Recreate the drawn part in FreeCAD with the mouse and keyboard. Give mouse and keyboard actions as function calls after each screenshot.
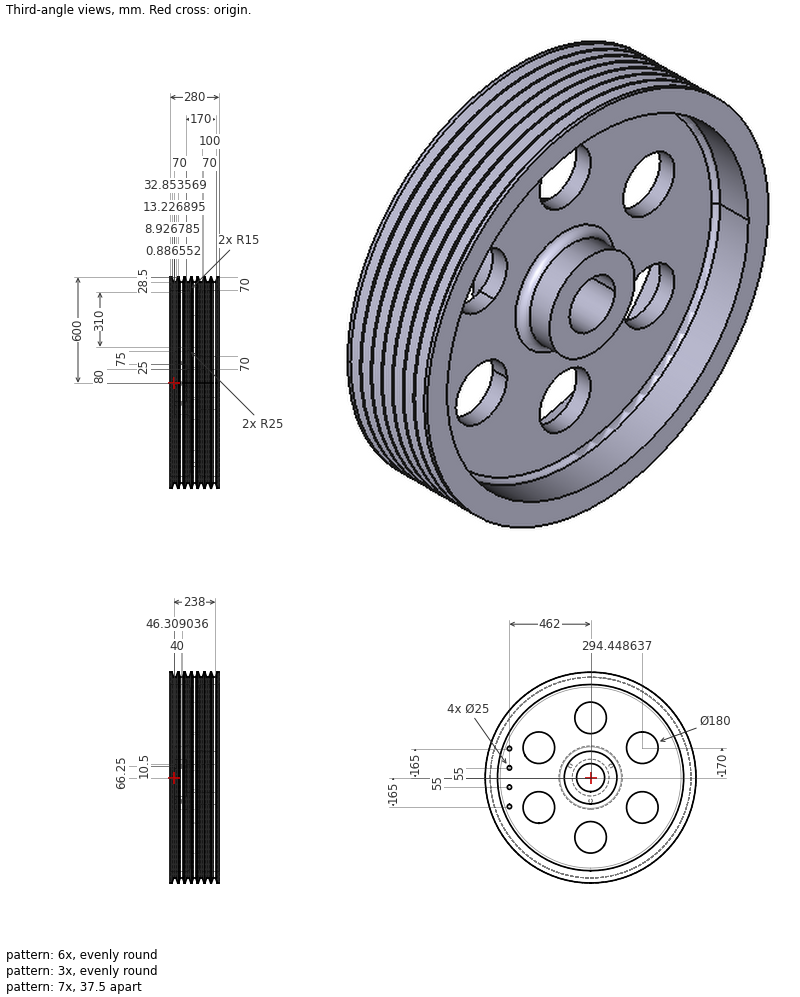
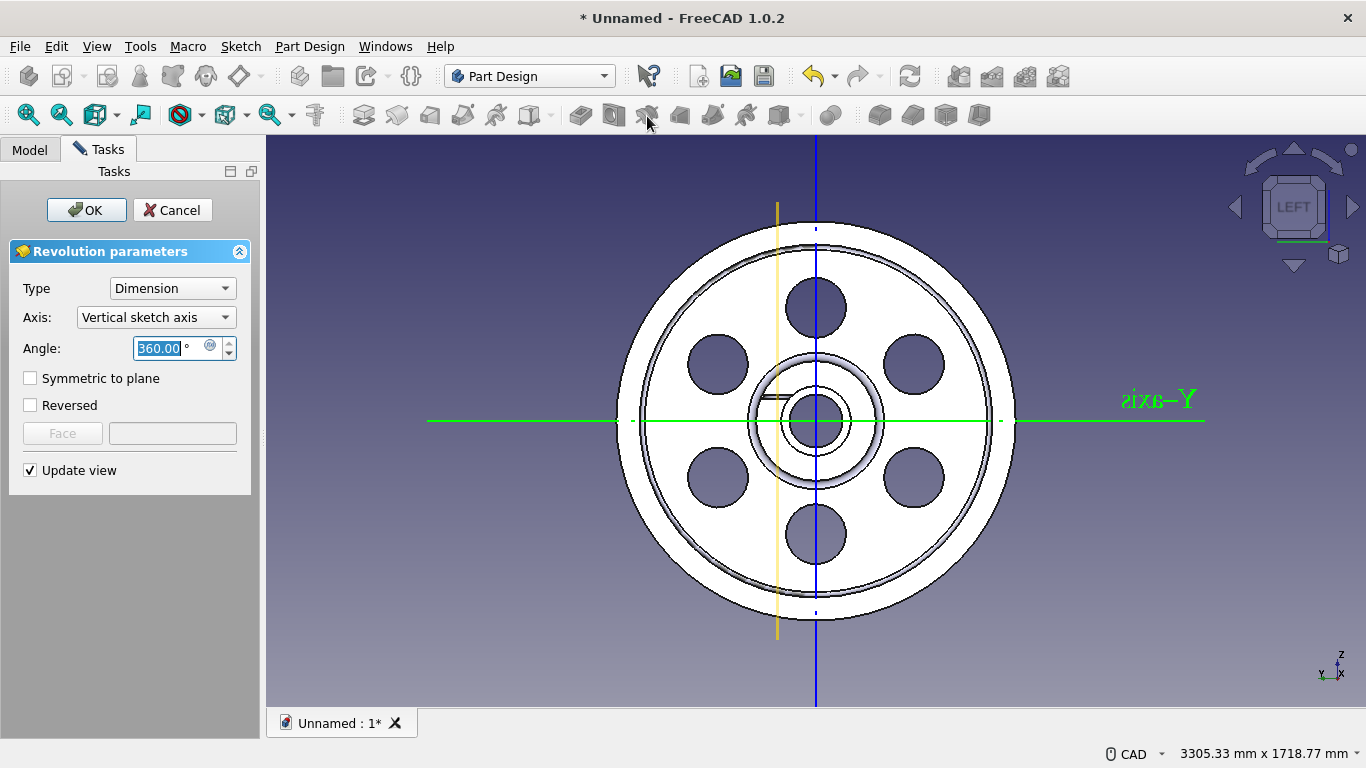
click(157, 318)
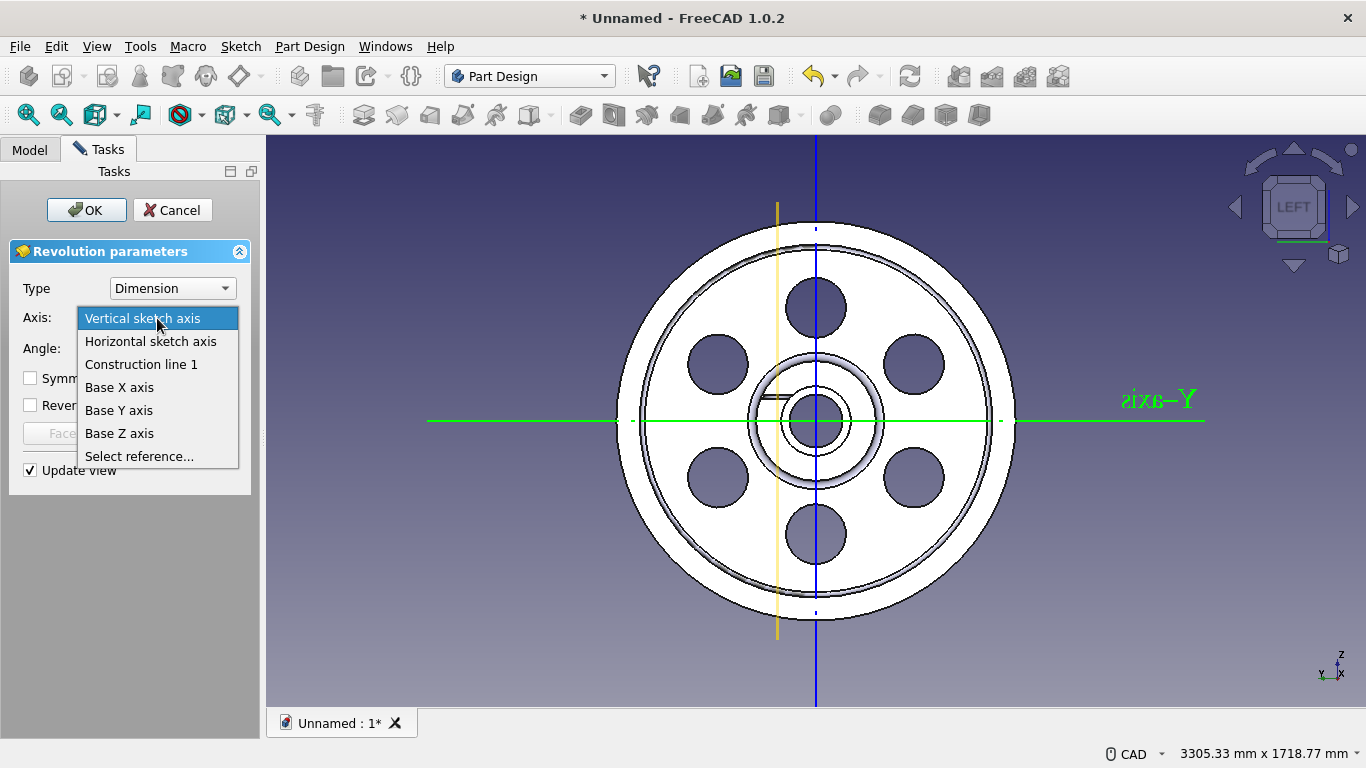
click(156, 364)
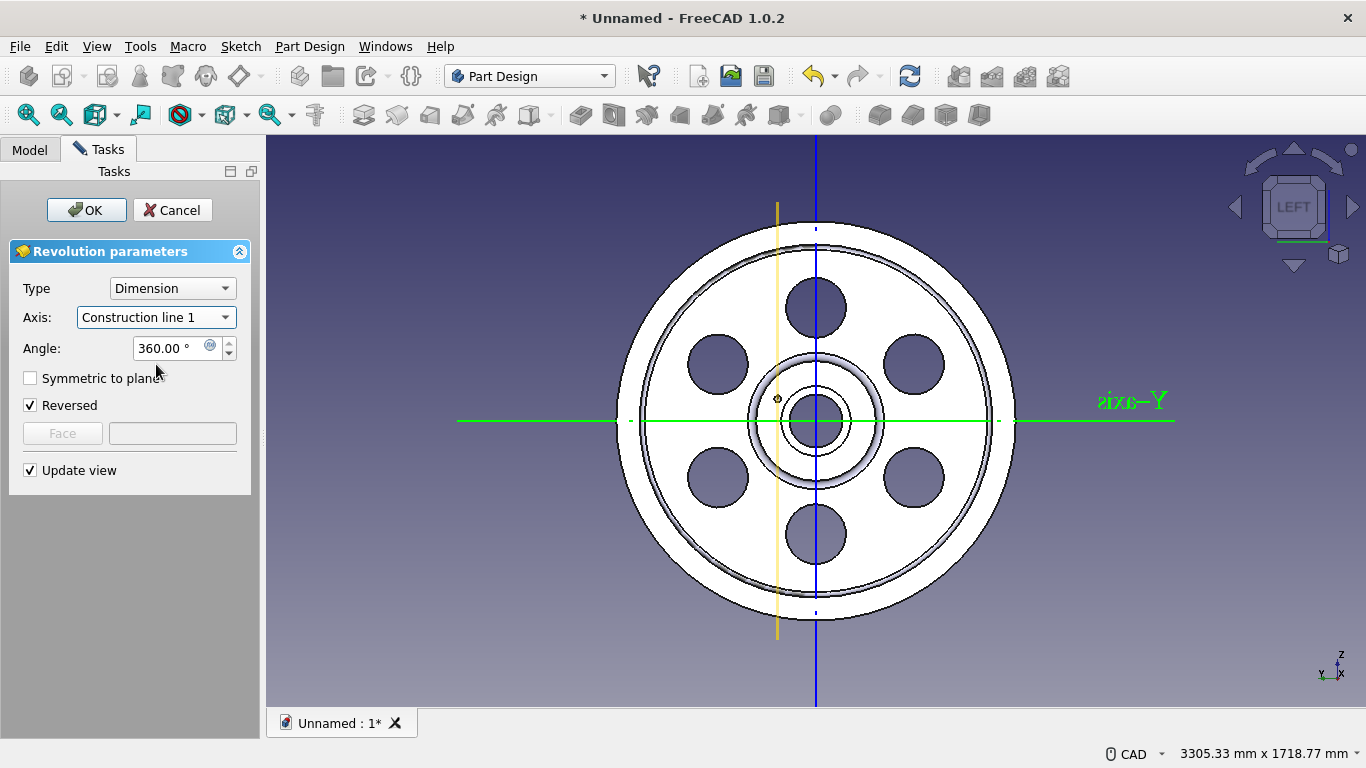
click(87, 210)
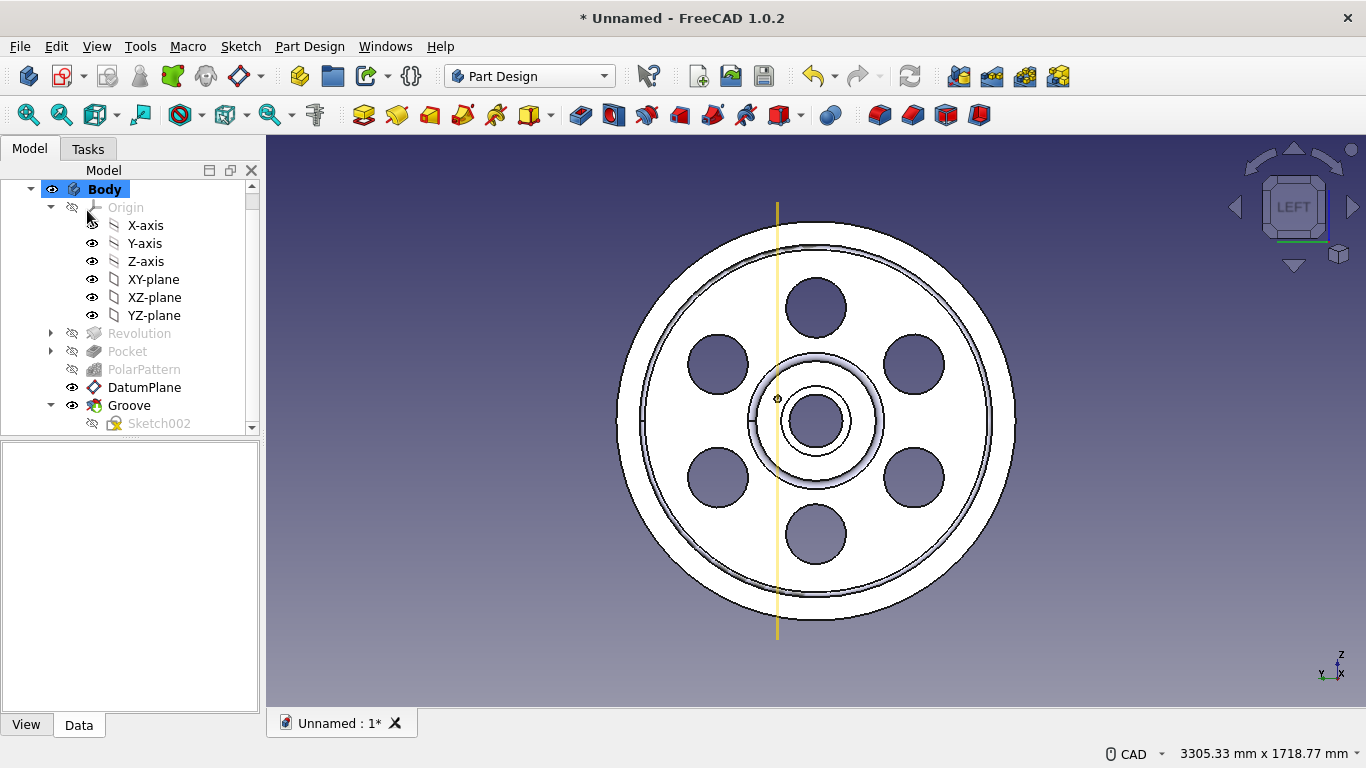
click(117, 387)
key(space)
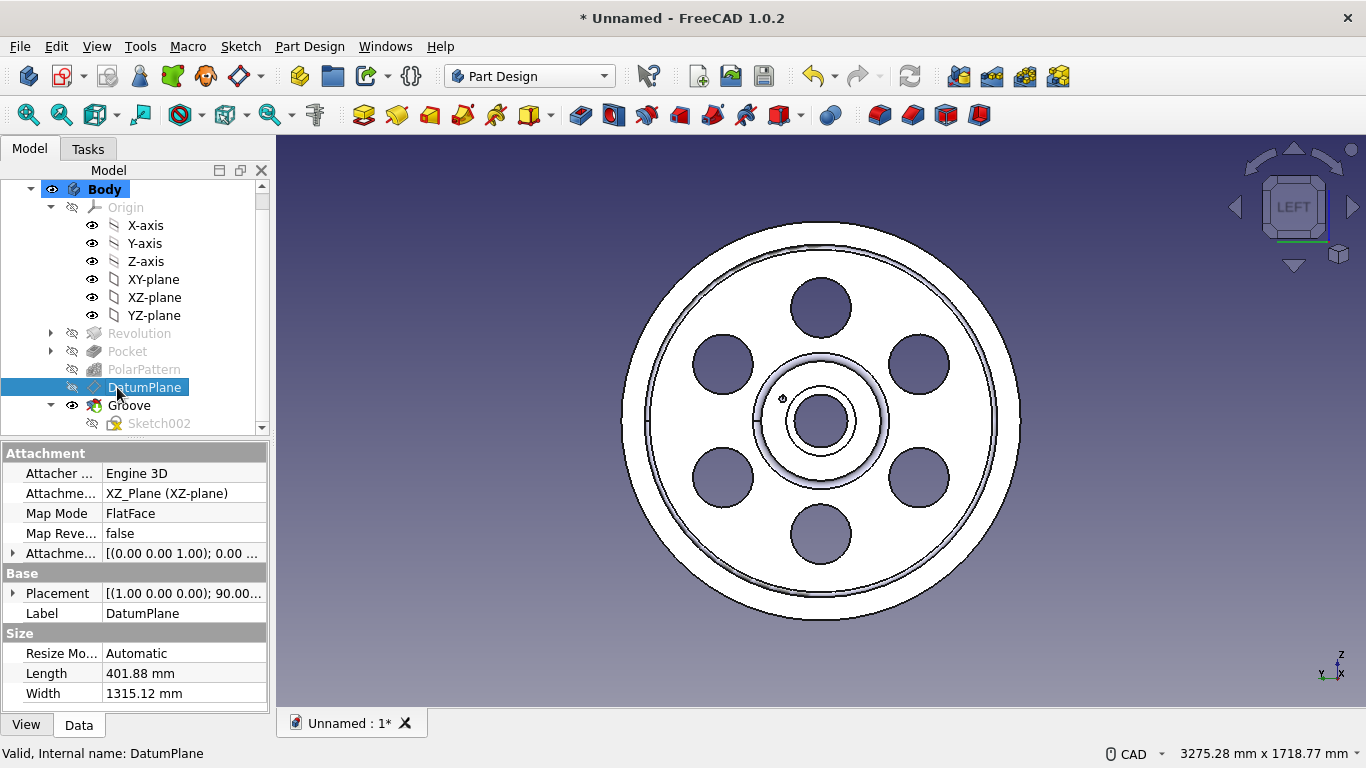
click(117, 405)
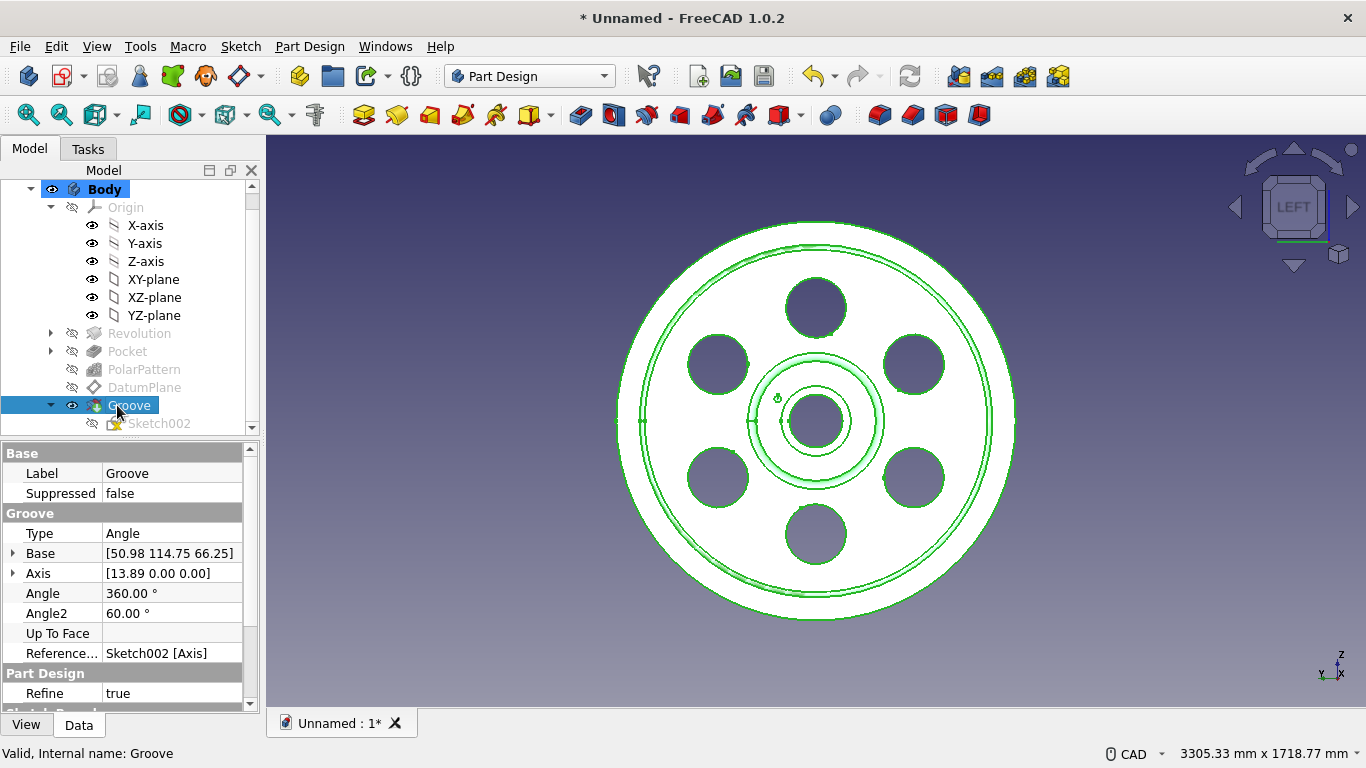
click(1025, 76)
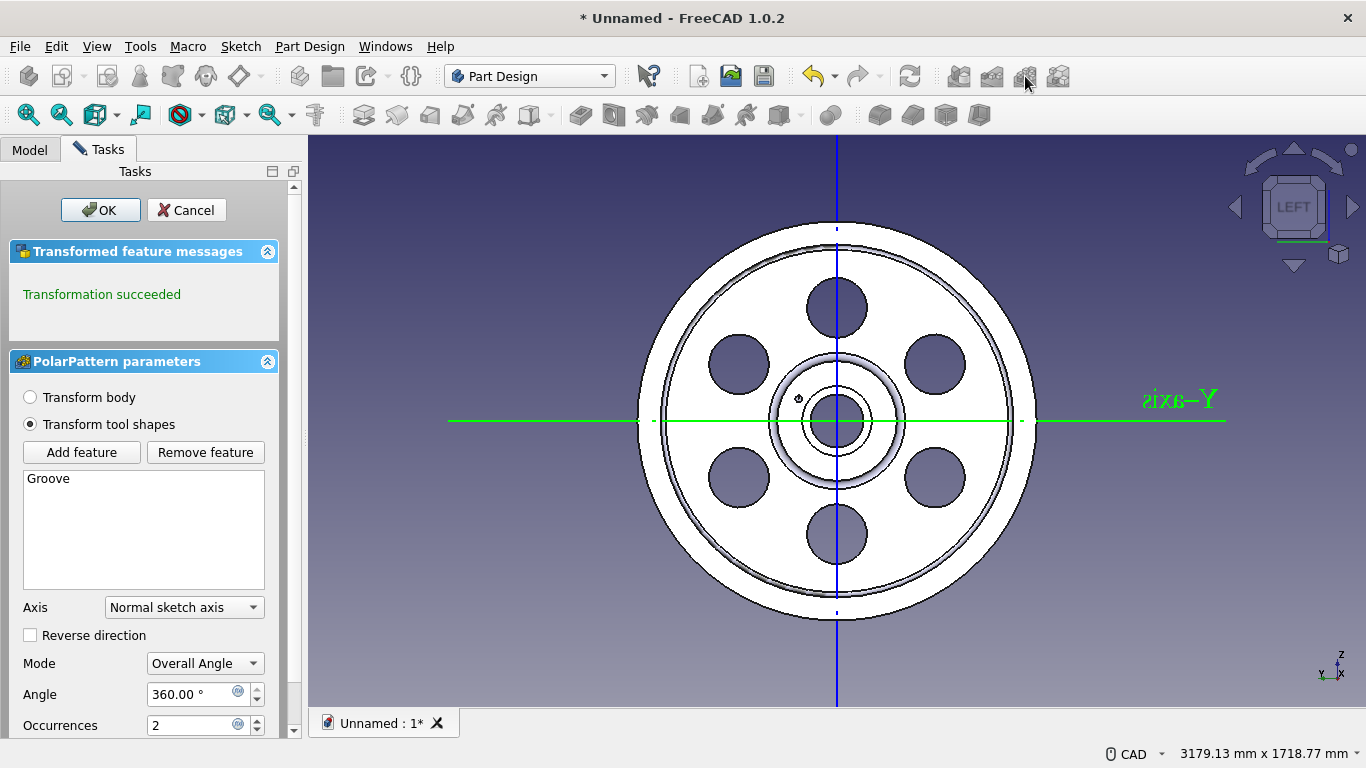
click(185, 608)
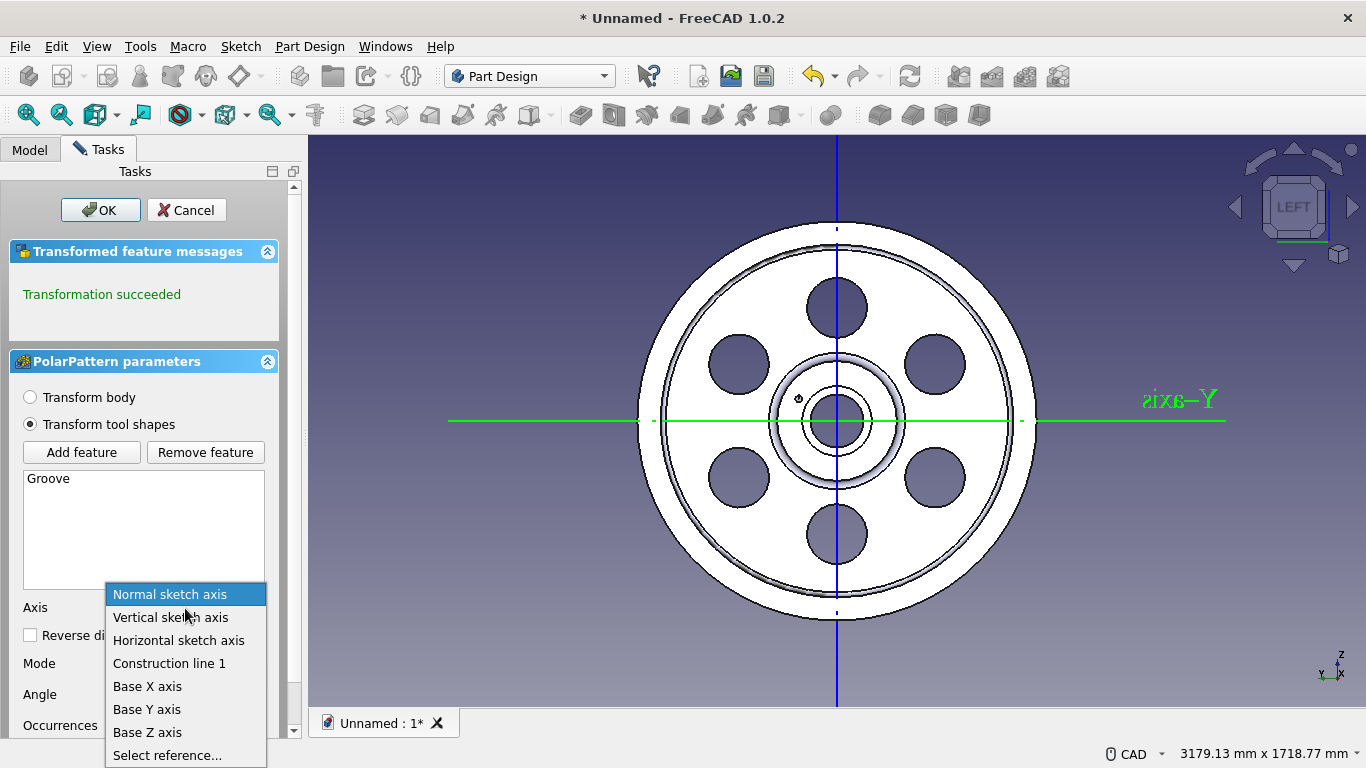
click(184, 686)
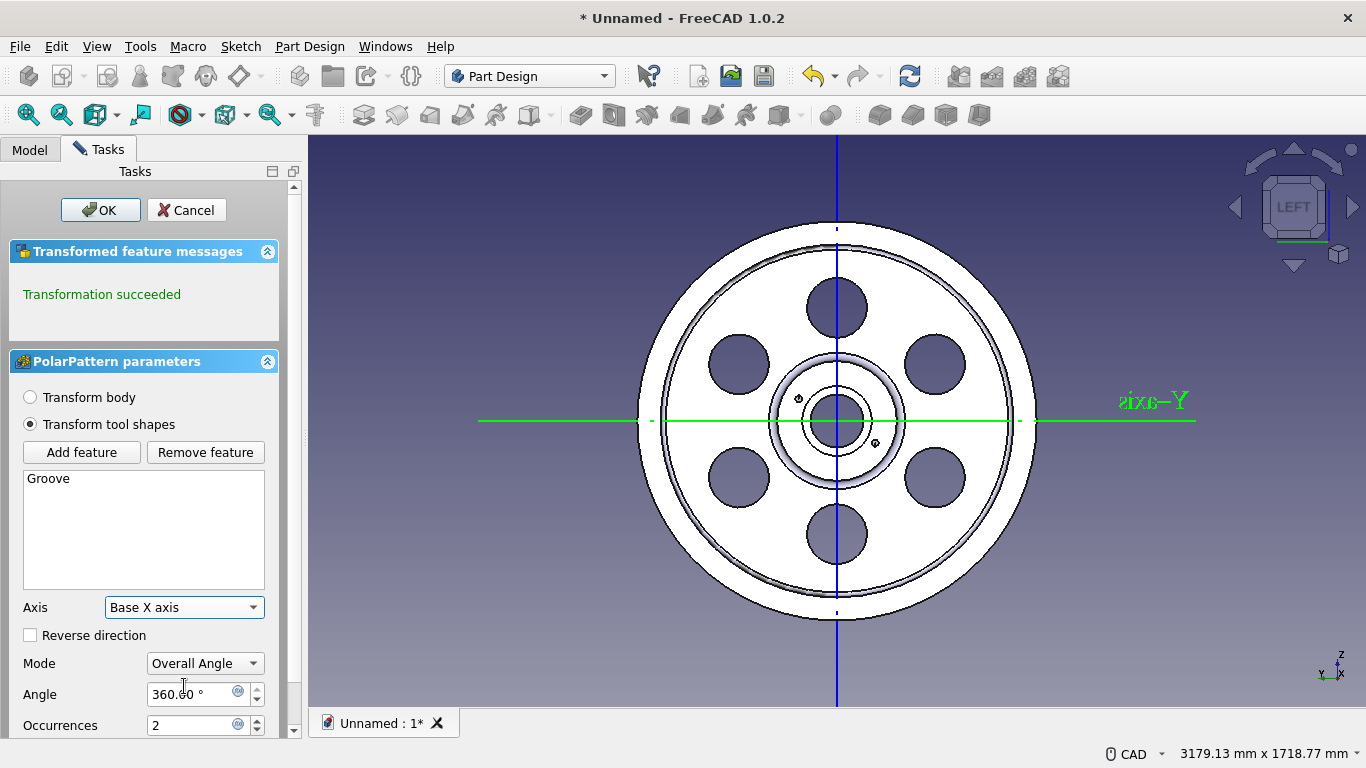
triple_click(199, 726)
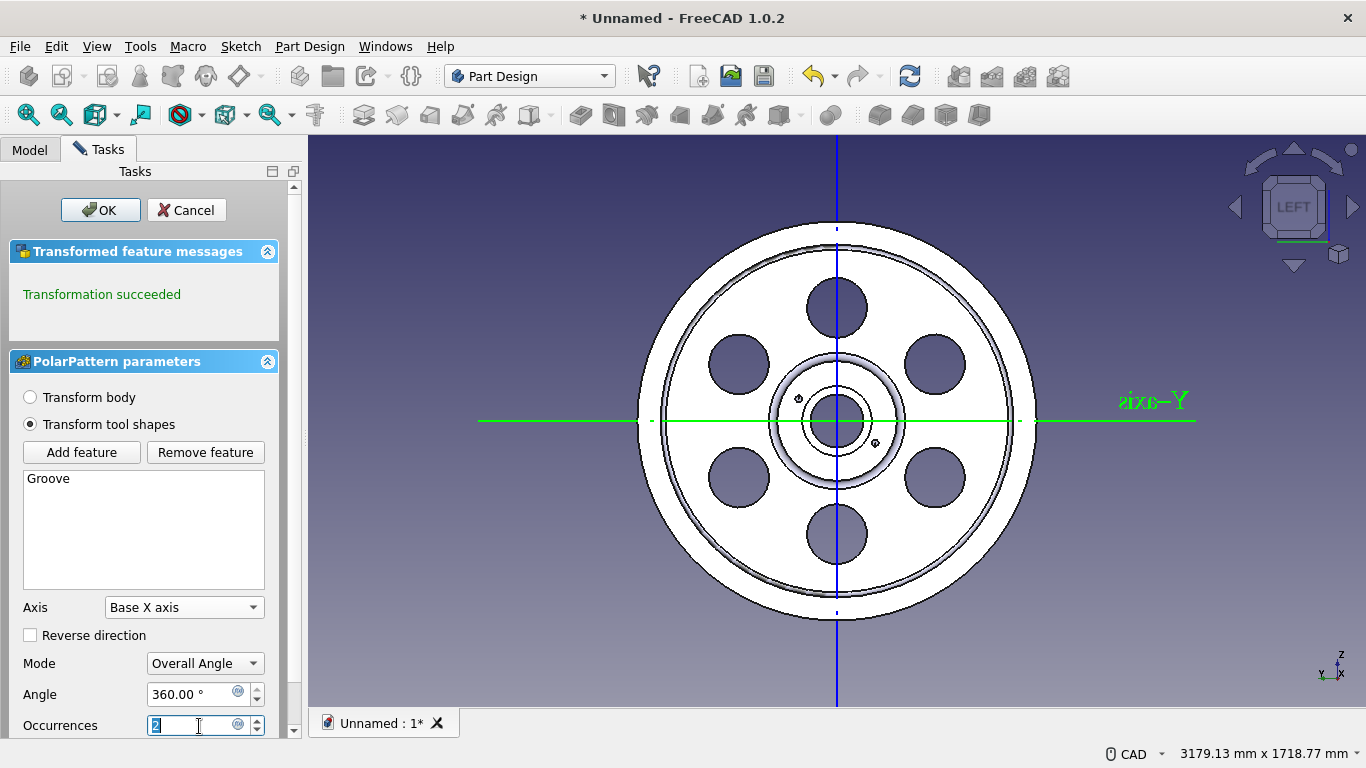
text(3)
key(Tab)